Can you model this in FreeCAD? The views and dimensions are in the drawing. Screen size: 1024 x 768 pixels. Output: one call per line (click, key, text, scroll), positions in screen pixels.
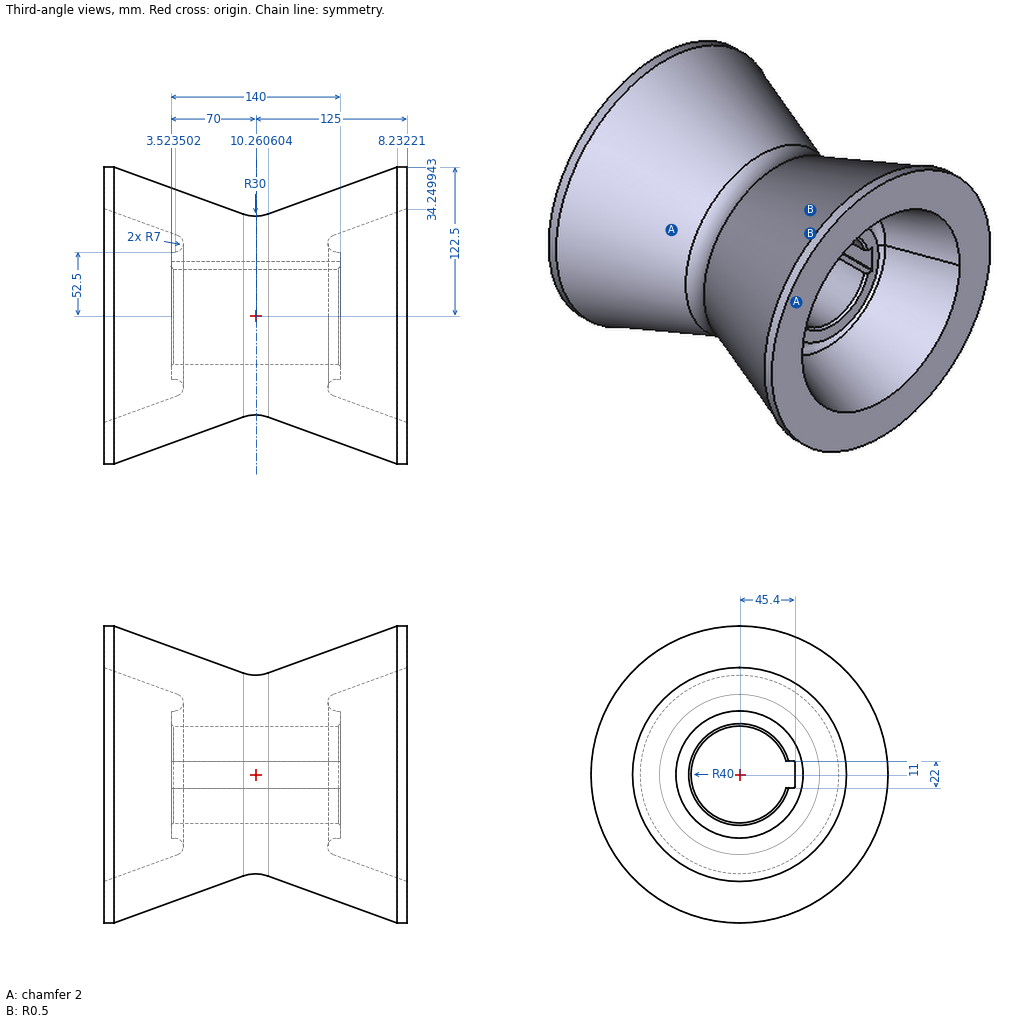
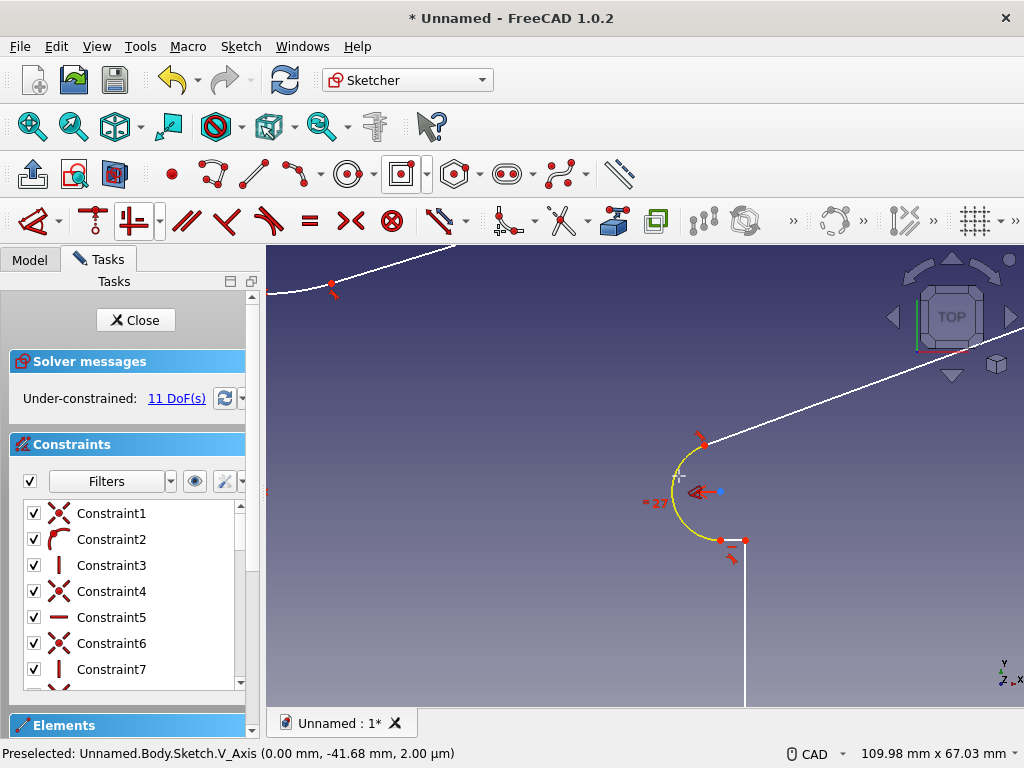
click(676, 474)
click(646, 462)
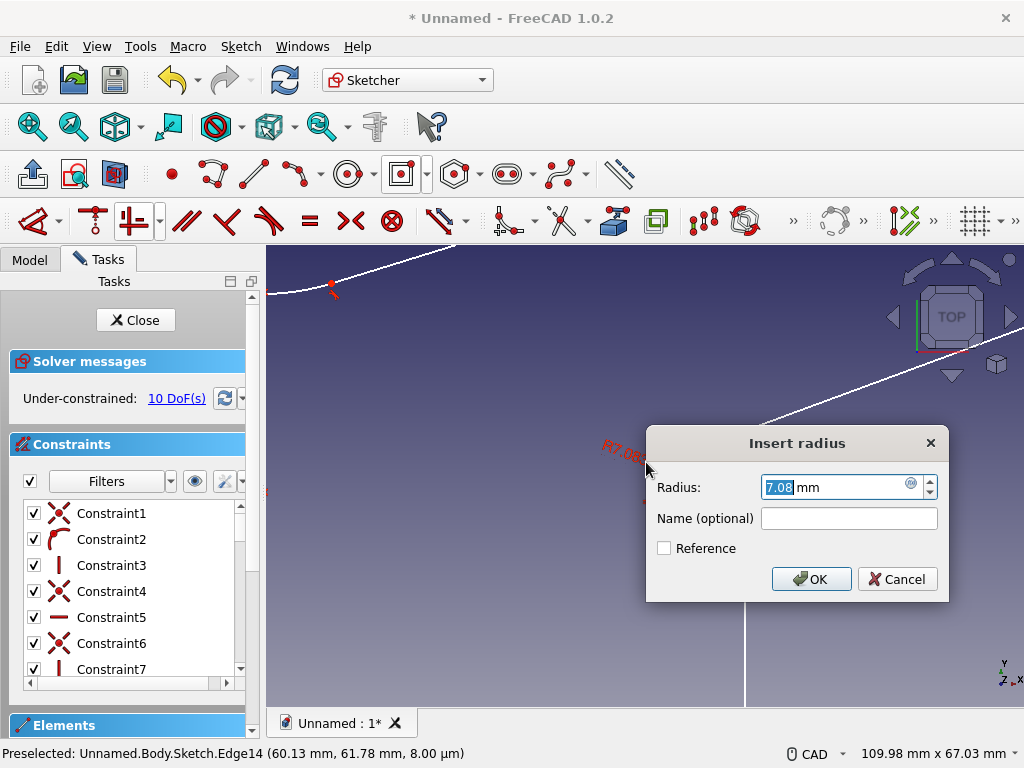
text(7)
key(Return)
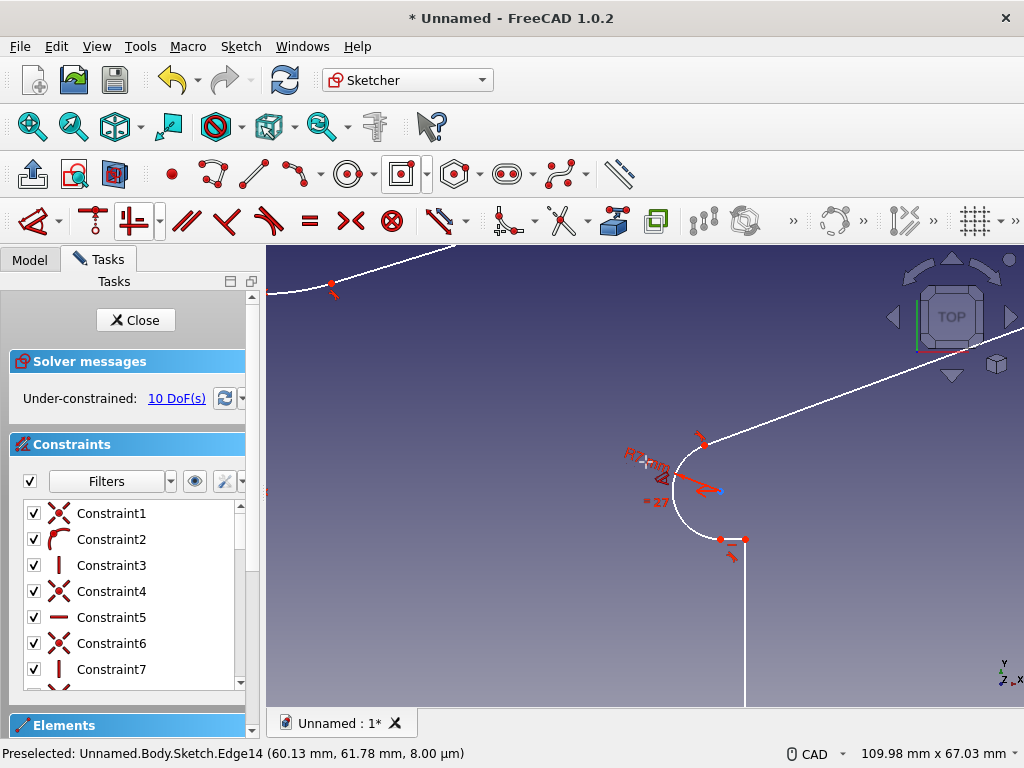
click(304, 290)
click(310, 321)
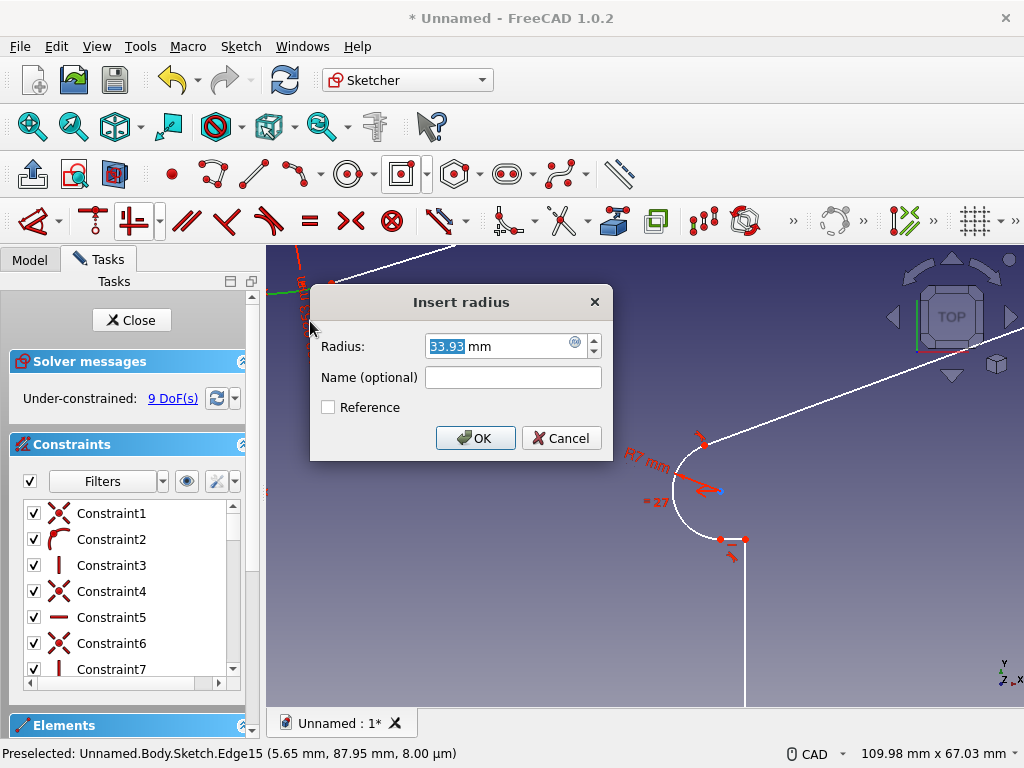
text(30)
key(Return)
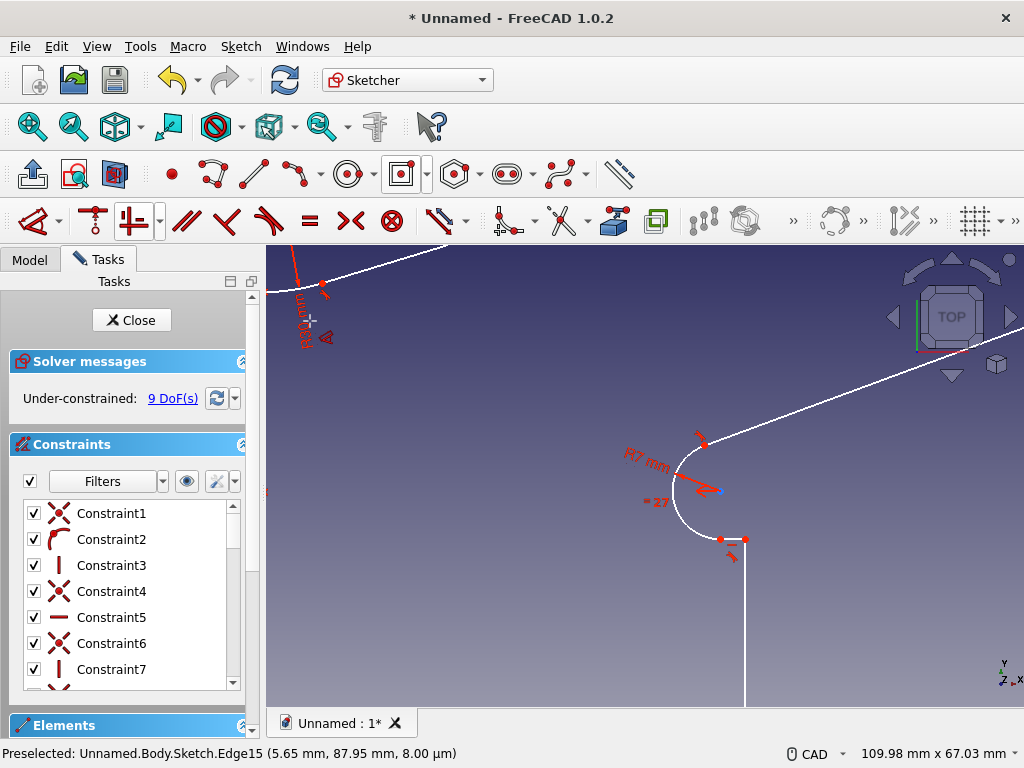
scroll(679, 476, down, 7)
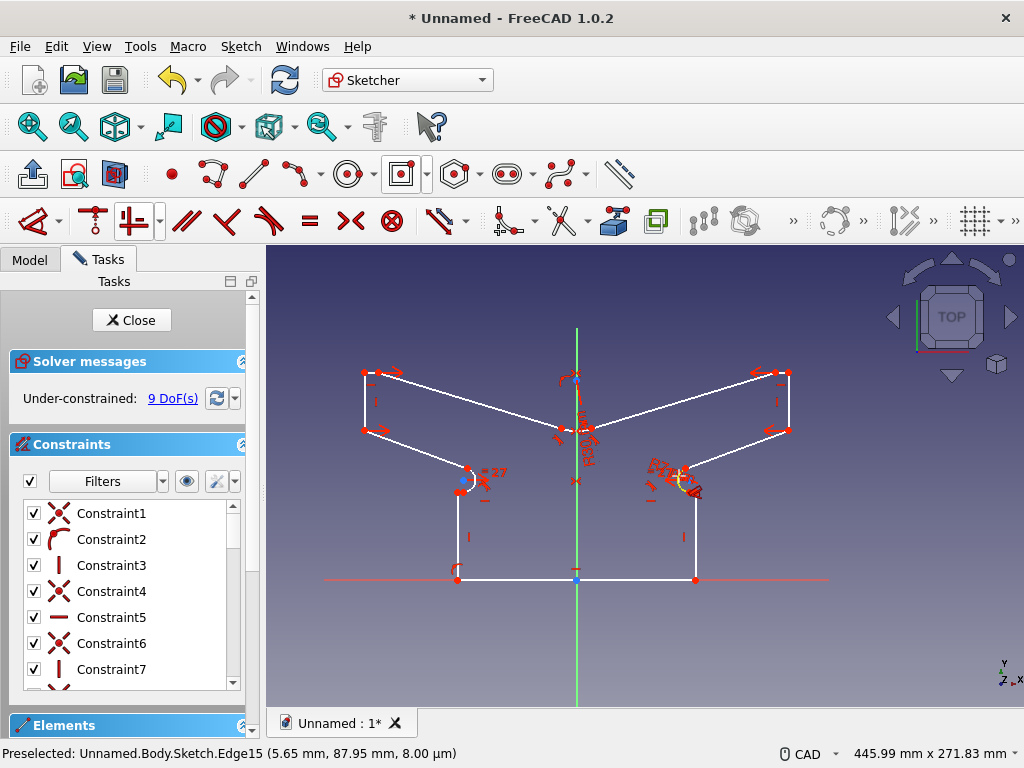
click(529, 580)
click(522, 614)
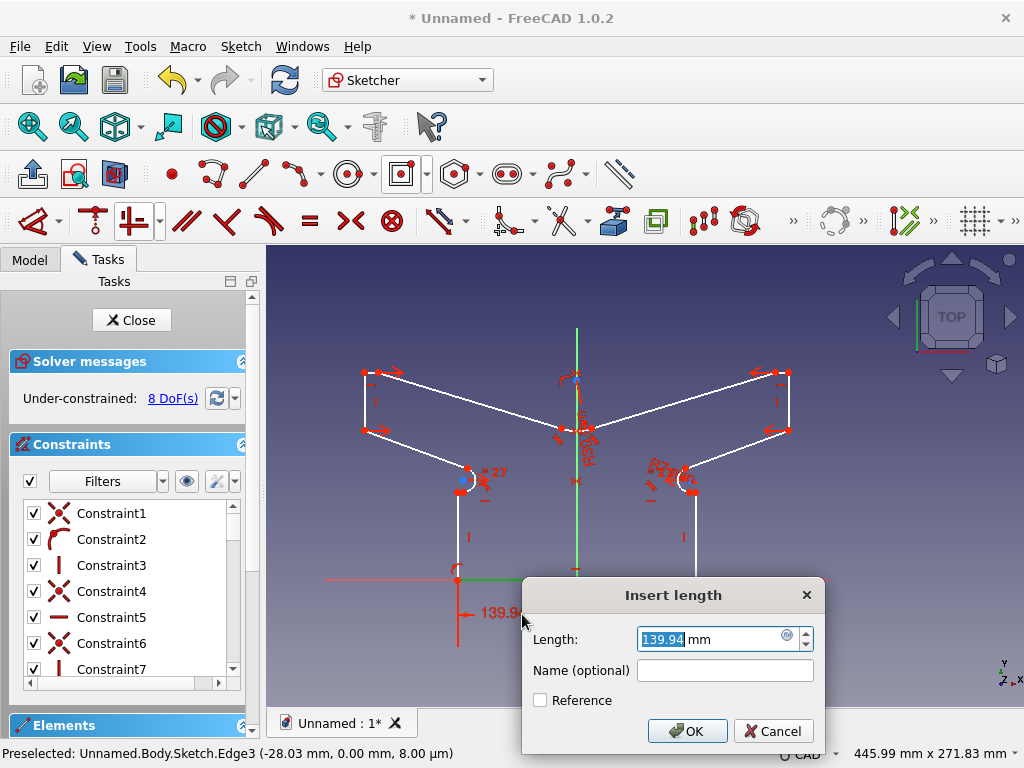
text(140)
key(Return)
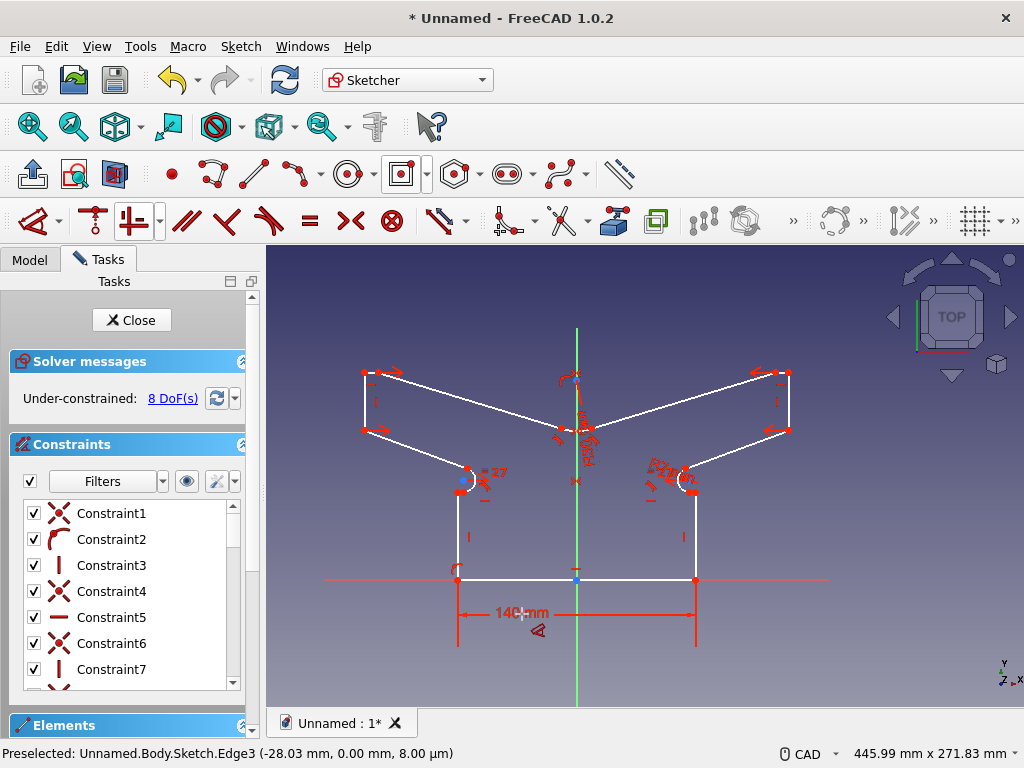
scroll(458, 492, up, 4)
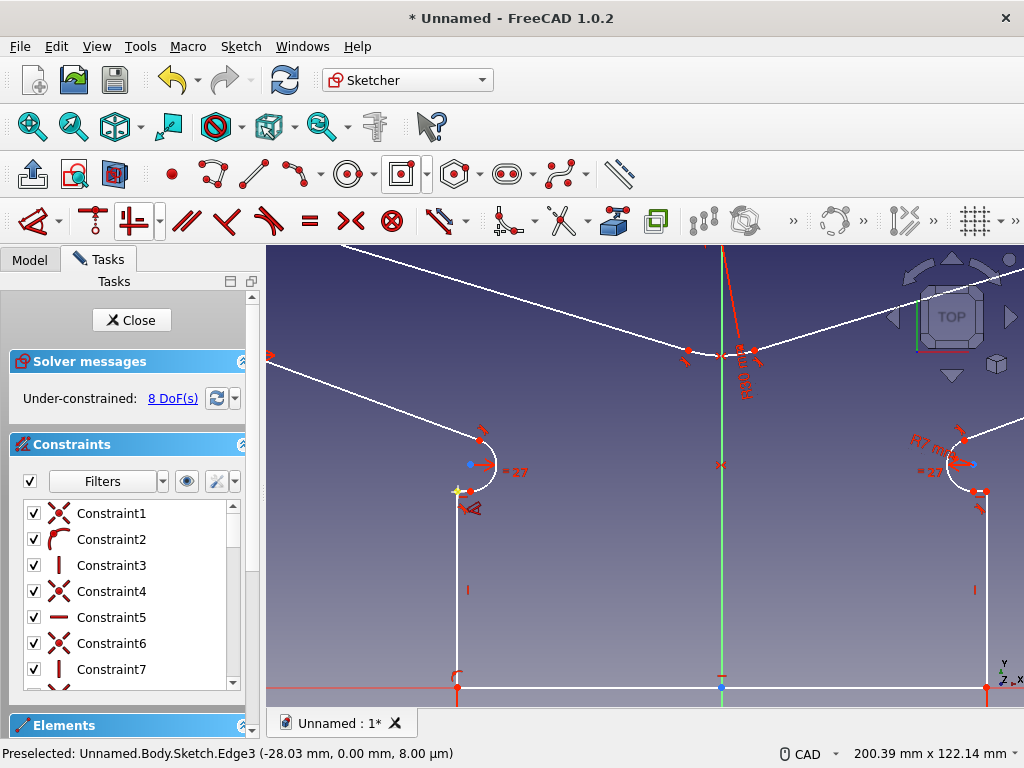
click(457, 491)
click(590, 457)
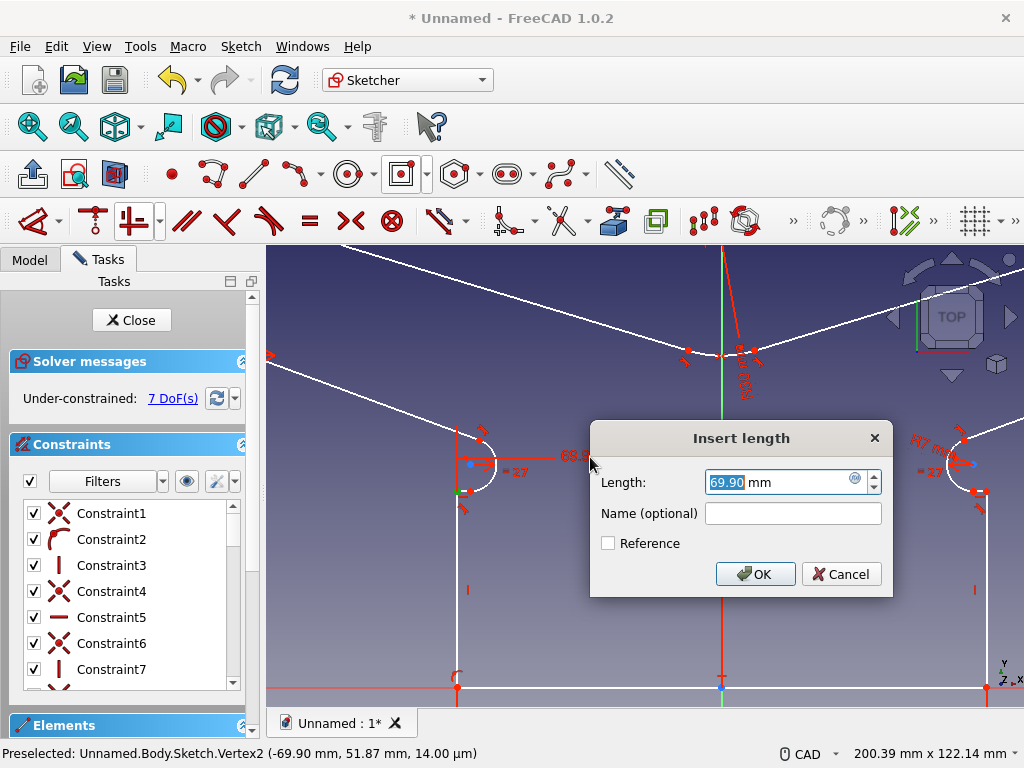
text(70)
key(Return)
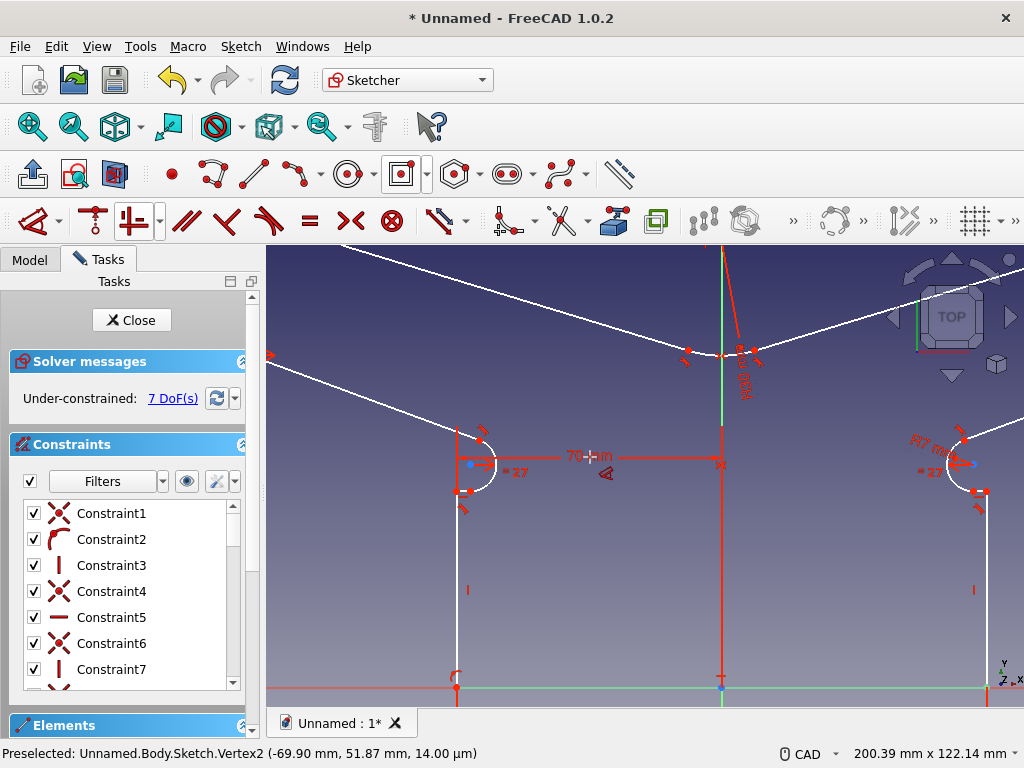
click(457, 550)
click(423, 585)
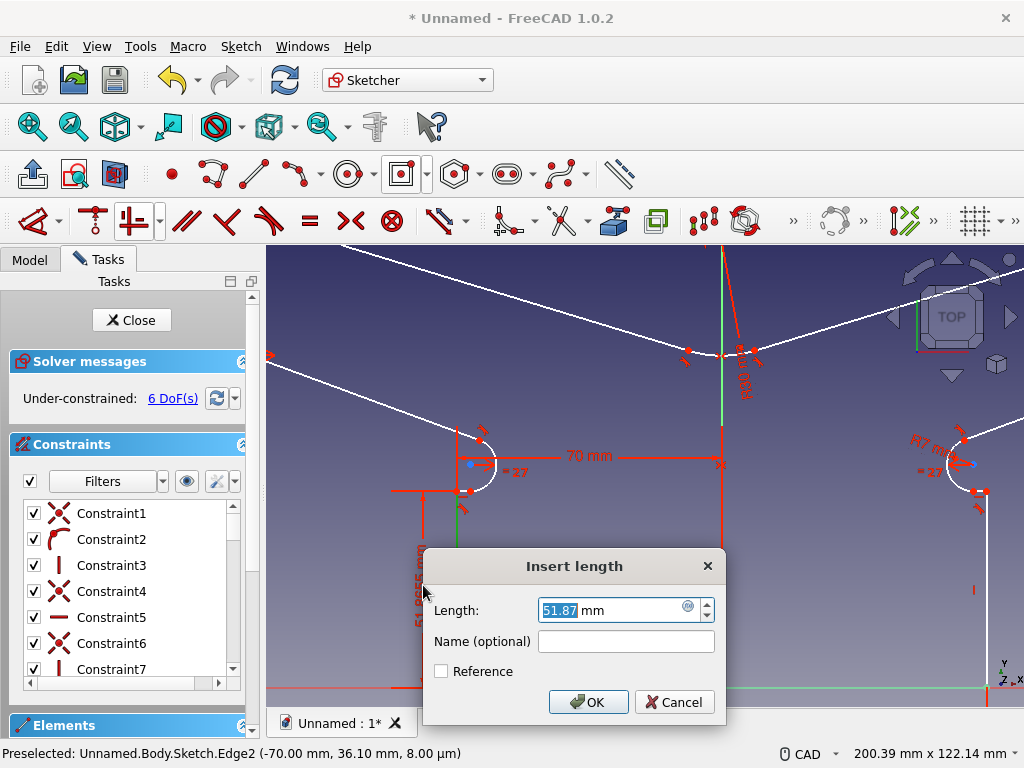
text(52.5)
key(Return)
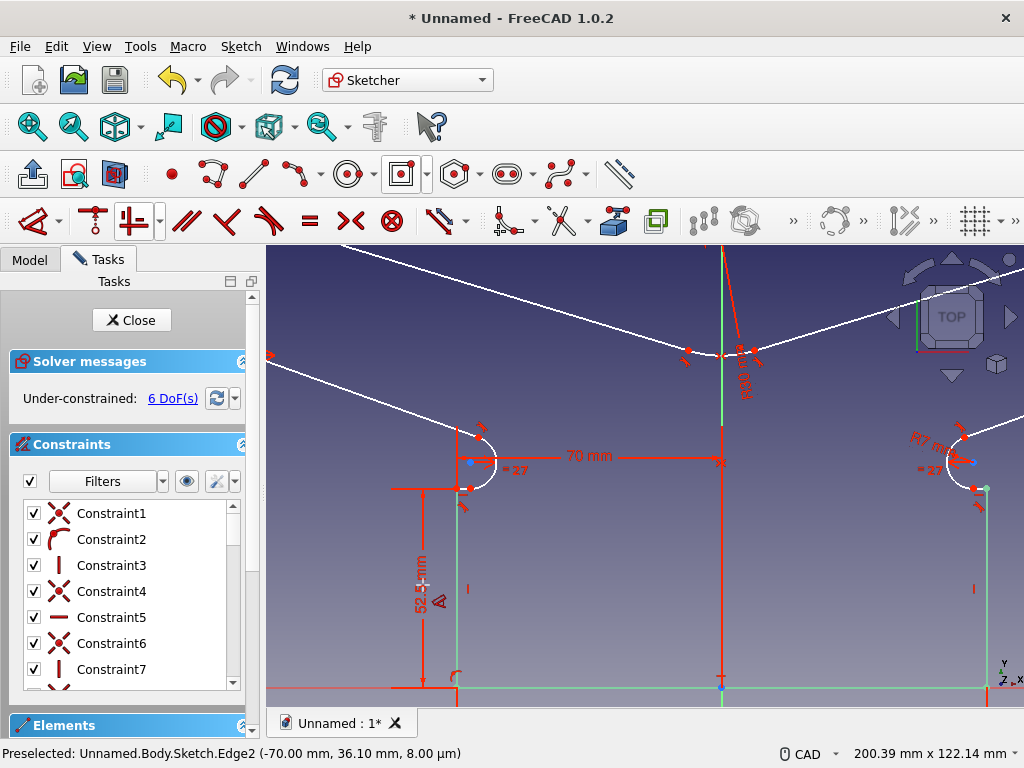
scroll(458, 492, down, 4)